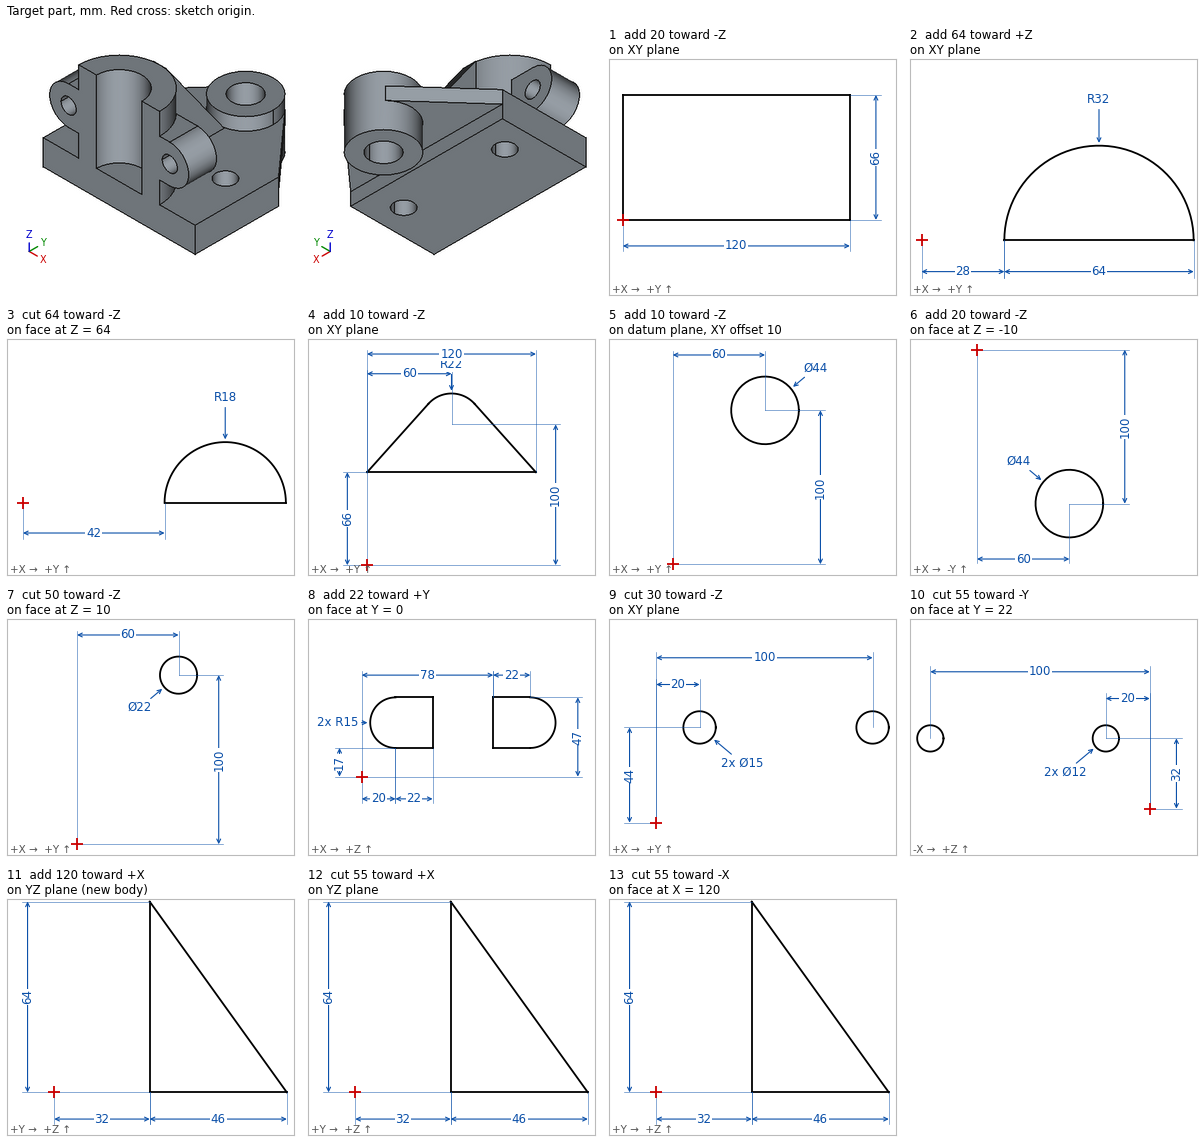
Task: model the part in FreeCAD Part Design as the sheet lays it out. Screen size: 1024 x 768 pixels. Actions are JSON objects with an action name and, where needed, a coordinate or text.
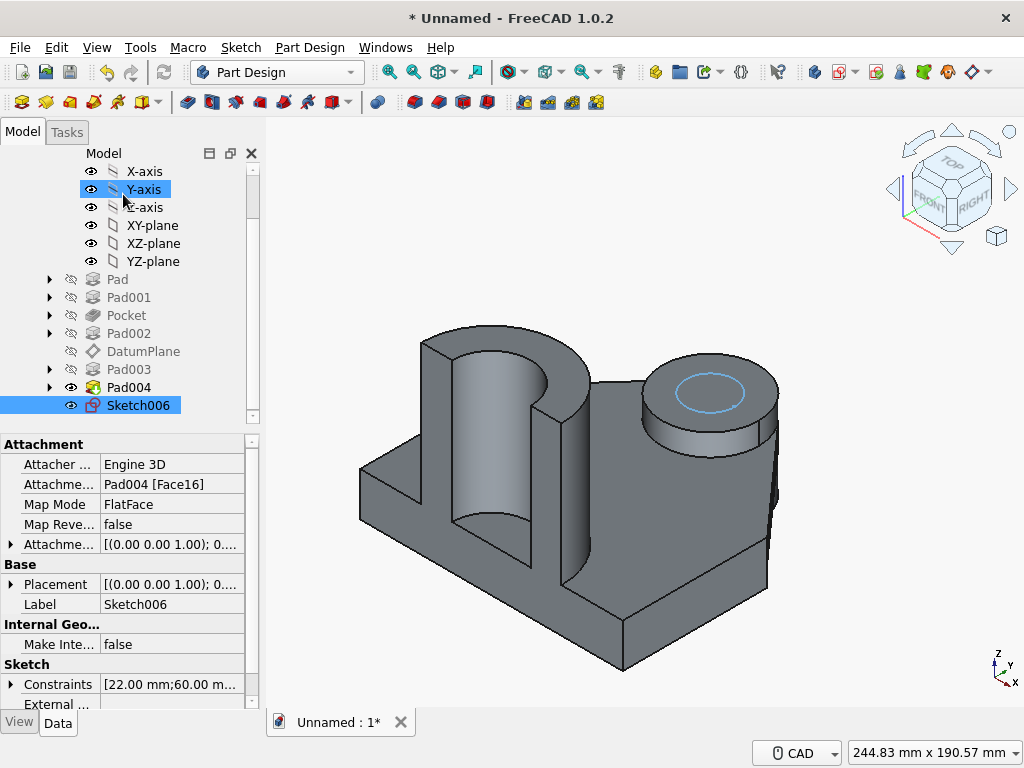
{"action": "left_click", "coordinate": [188, 102]}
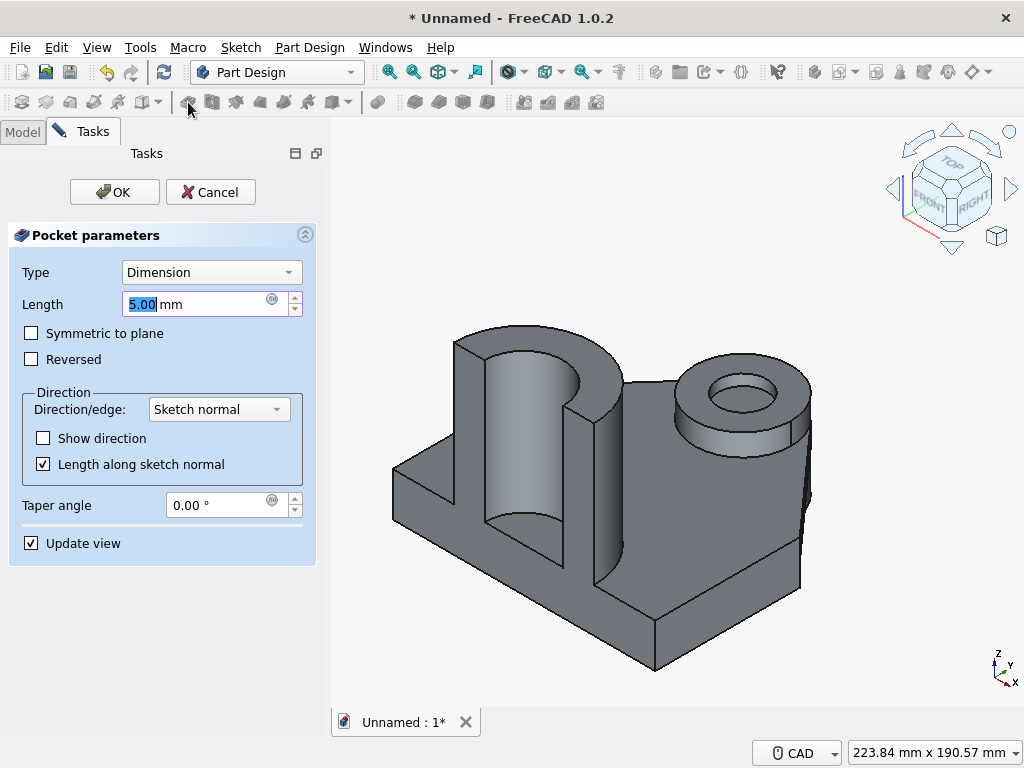
{"action": "type", "text": "50"}
{"action": "key", "text": "Tab"}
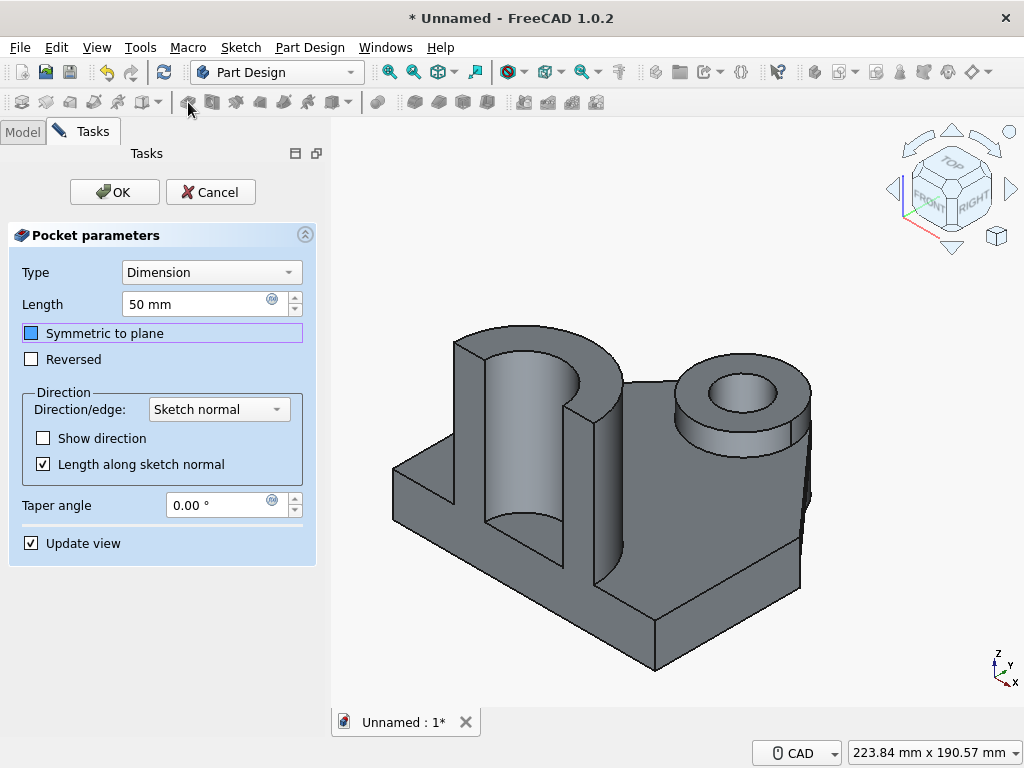
{"action": "left_click", "coordinate": [115, 192]}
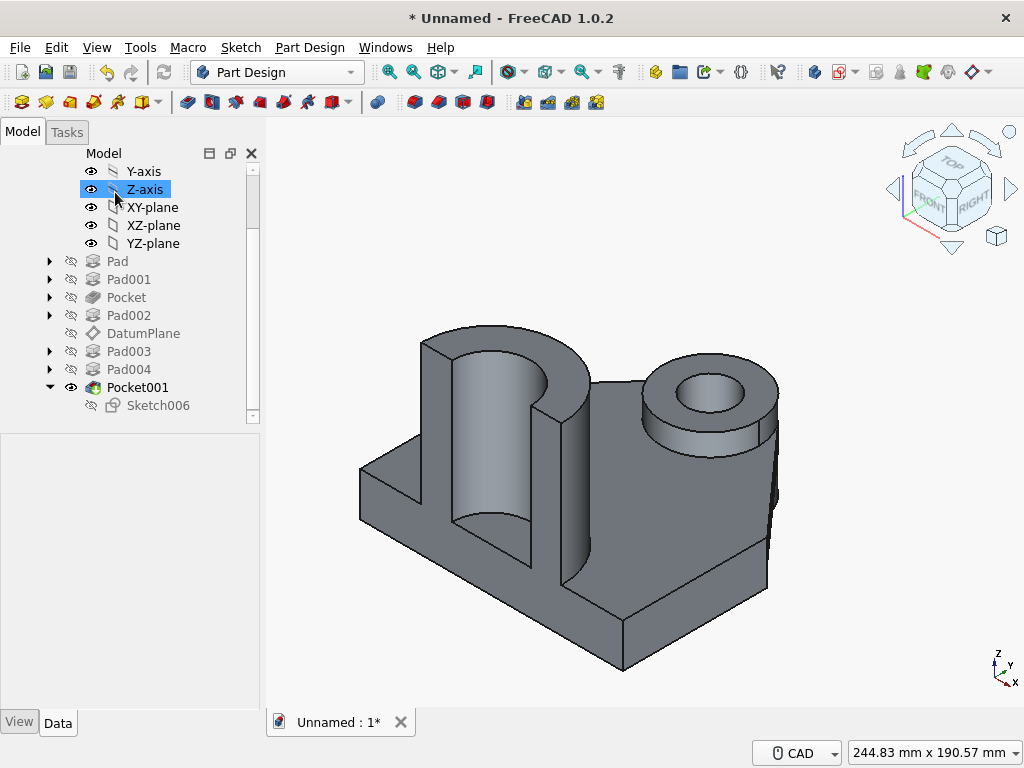
{"action": "left_click", "coordinate": [604, 644]}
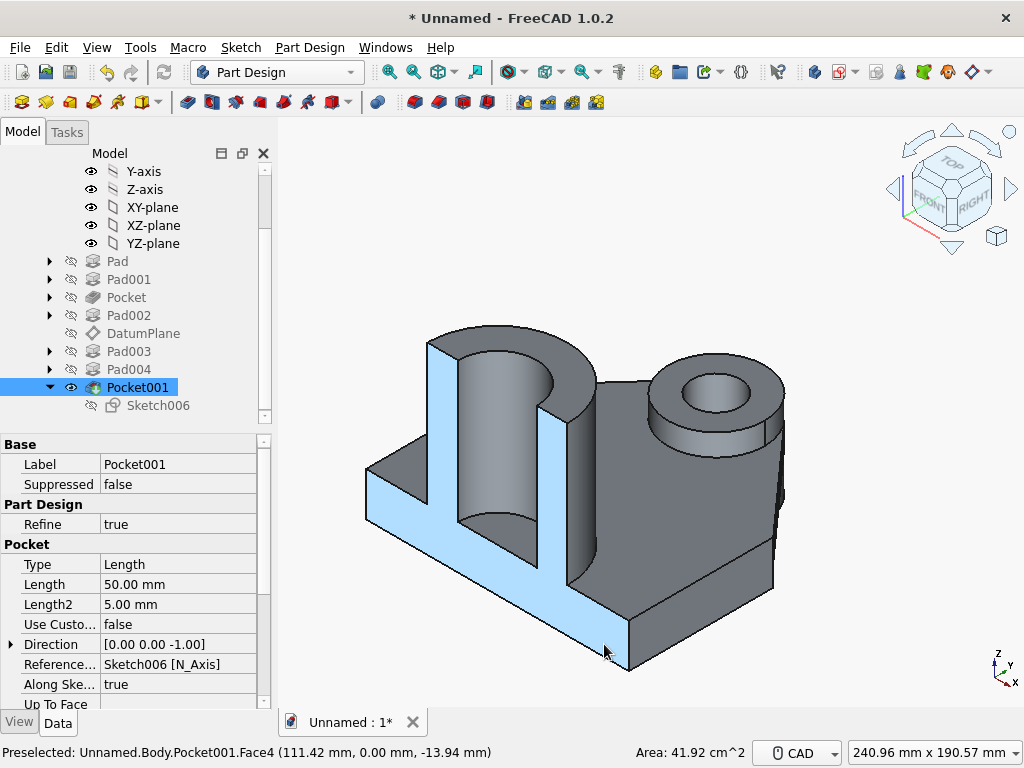
{"action": "left_click", "coordinate": [840, 72]}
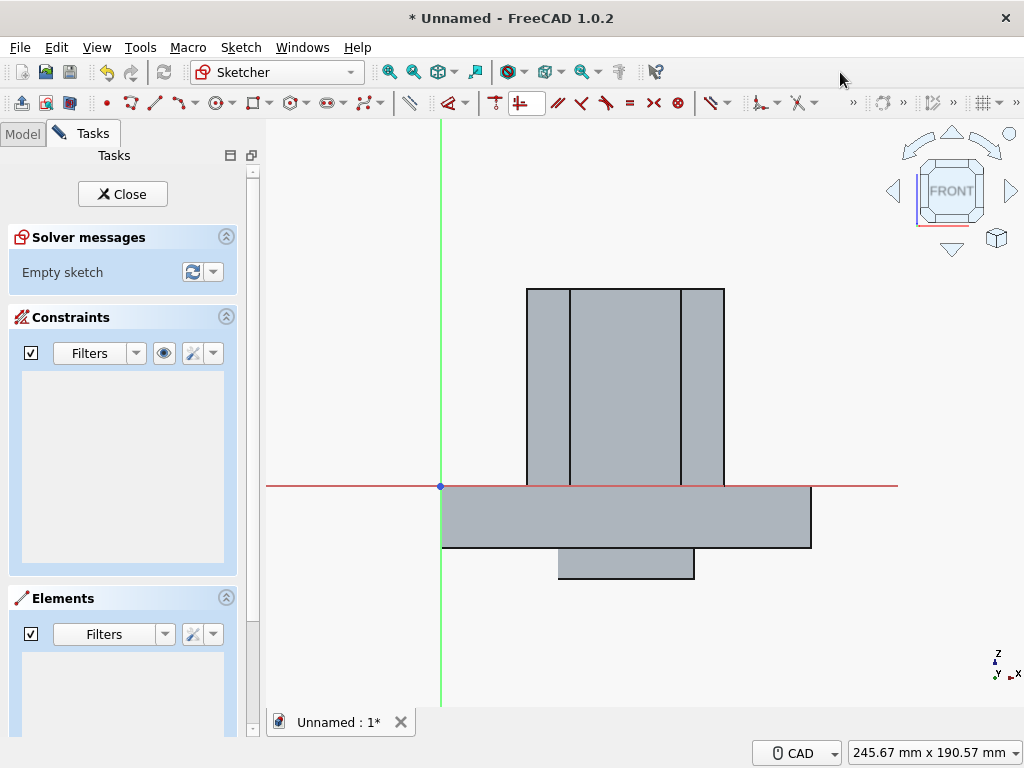
{"action": "left_click", "coordinate": [132, 104]}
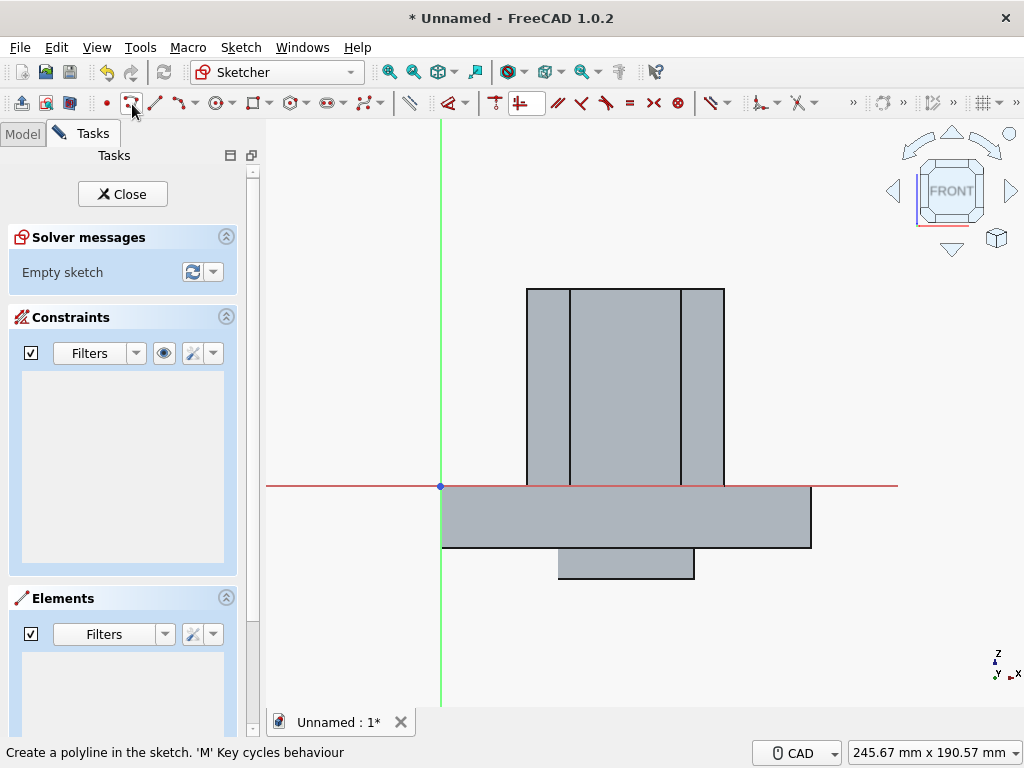
{"action": "left_click", "coordinate": [502, 434]}
{"action": "left_click", "coordinate": [570, 434]}
{"action": "left_click", "coordinate": [570, 341]}
{"action": "left_click", "coordinate": [502, 341]}
{"action": "right_click", "coordinate": [502, 341]}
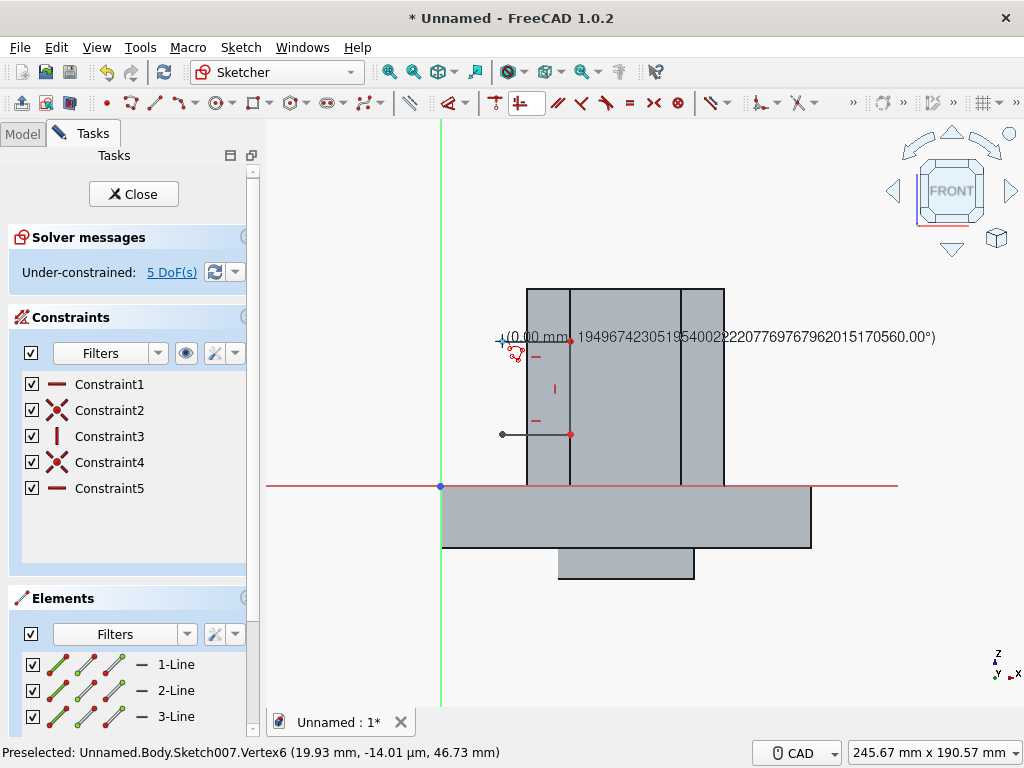
{"action": "left_click", "coordinate": [180, 104]}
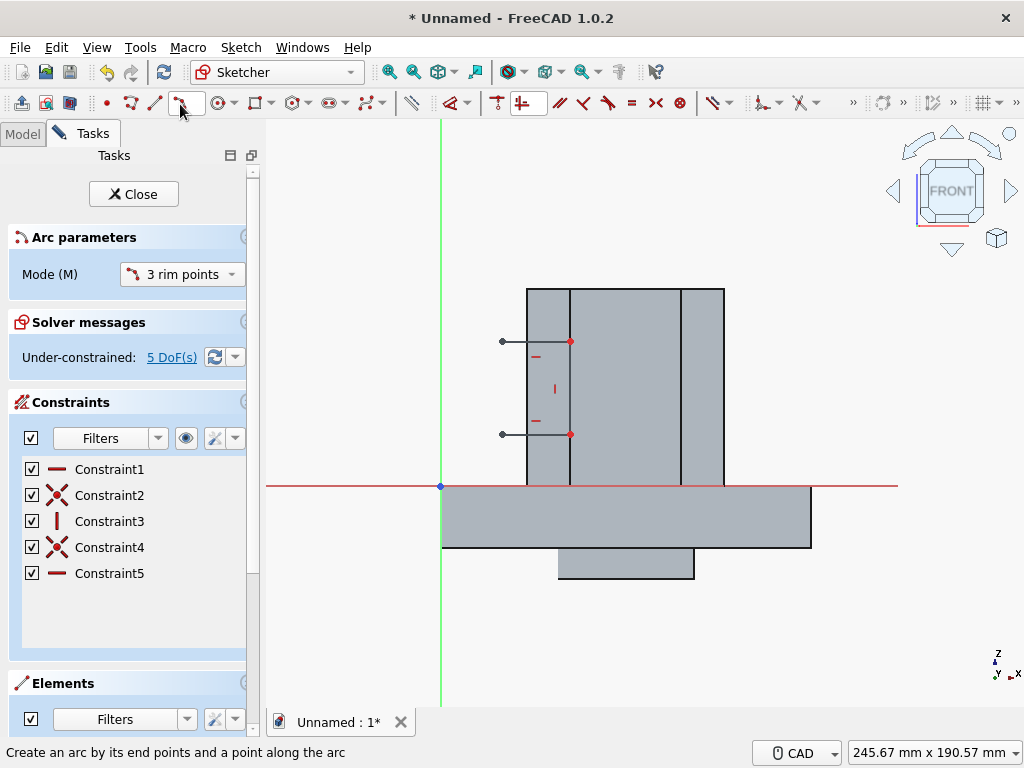
{"action": "left_click", "coordinate": [502, 342]}
{"action": "left_click", "coordinate": [502, 435]}
{"action": "left_click", "coordinate": [456, 387]}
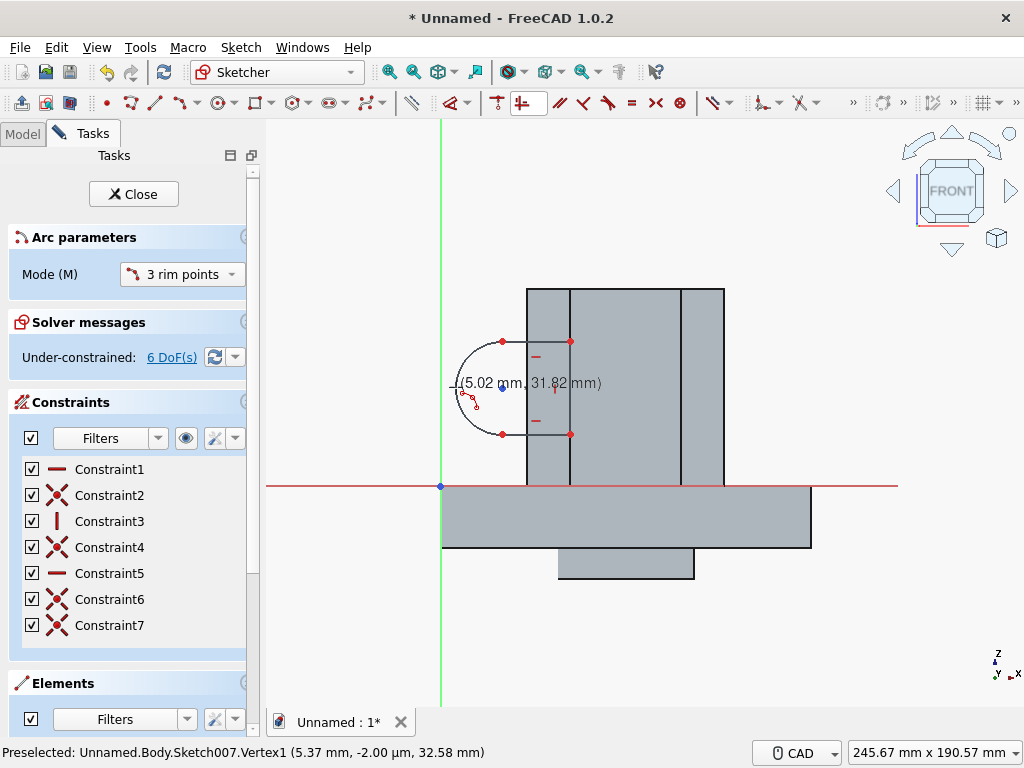
{"action": "left_click", "coordinate": [132, 104]}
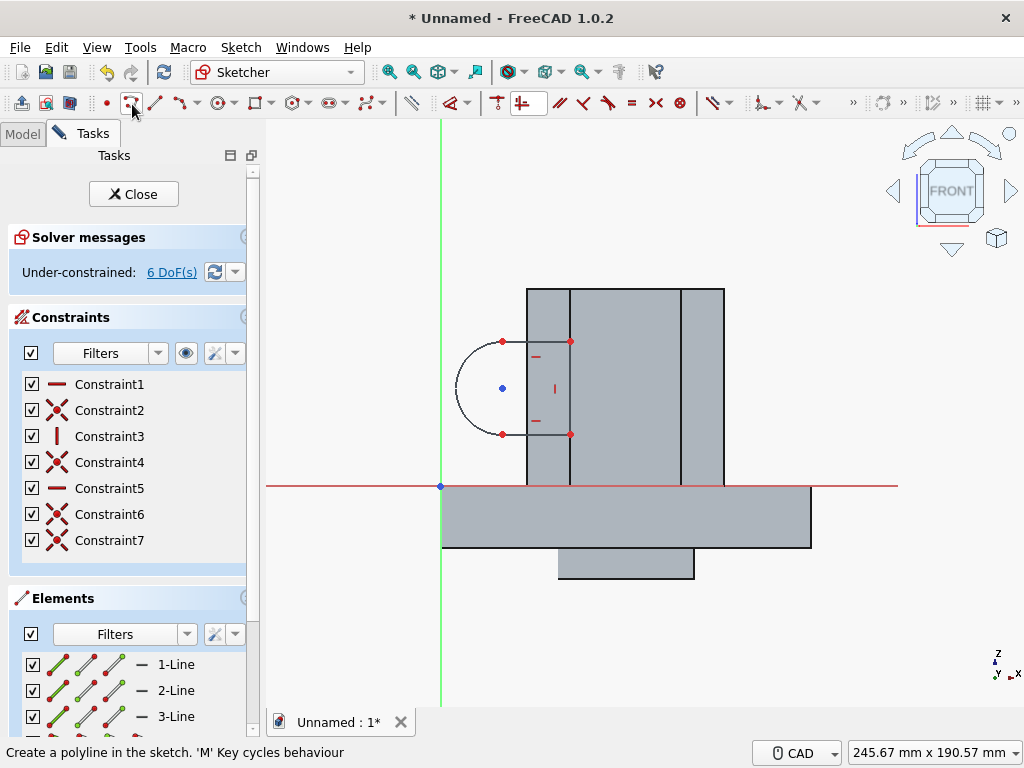
{"action": "left_click", "coordinate": [749, 341]}
{"action": "left_click", "coordinate": [681, 341]}
{"action": "left_click", "coordinate": [681, 434]}
{"action": "left_click", "coordinate": [749, 434]}
{"action": "right_click", "coordinate": [749, 434]}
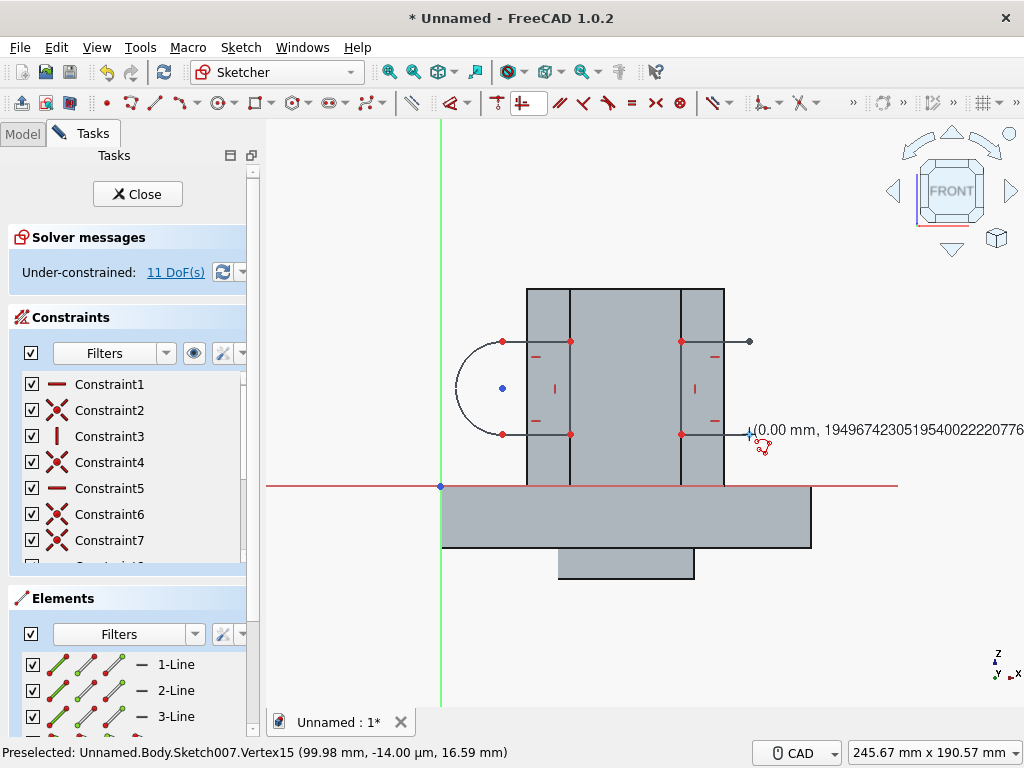
{"action": "left_click", "coordinate": [180, 104]}